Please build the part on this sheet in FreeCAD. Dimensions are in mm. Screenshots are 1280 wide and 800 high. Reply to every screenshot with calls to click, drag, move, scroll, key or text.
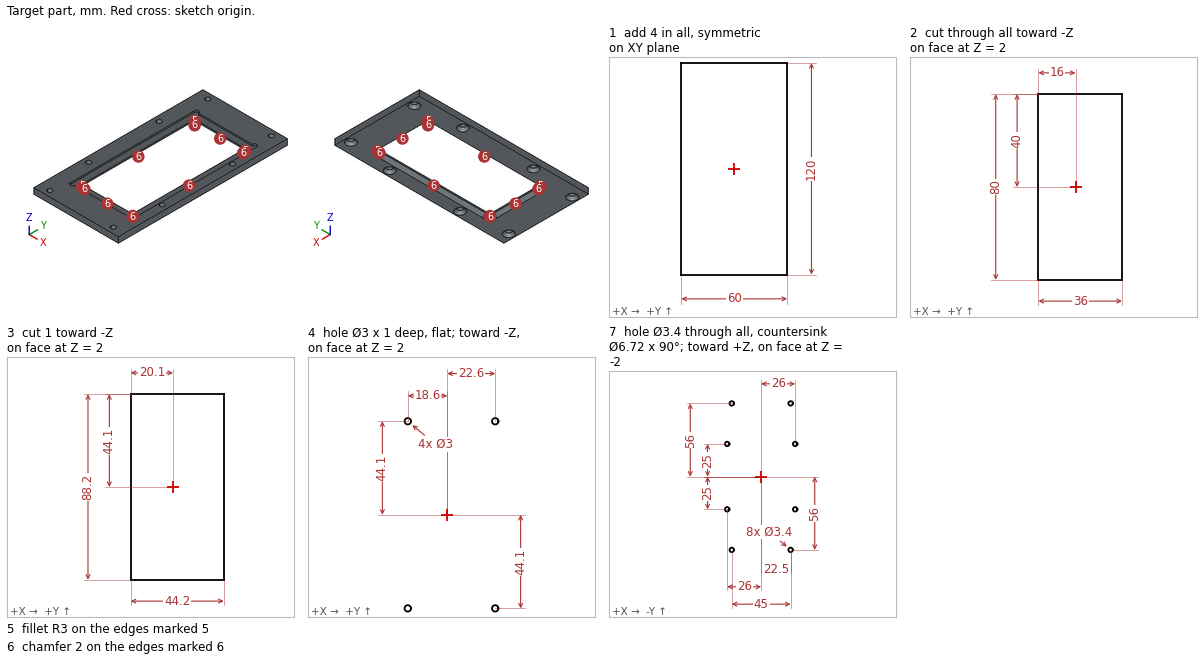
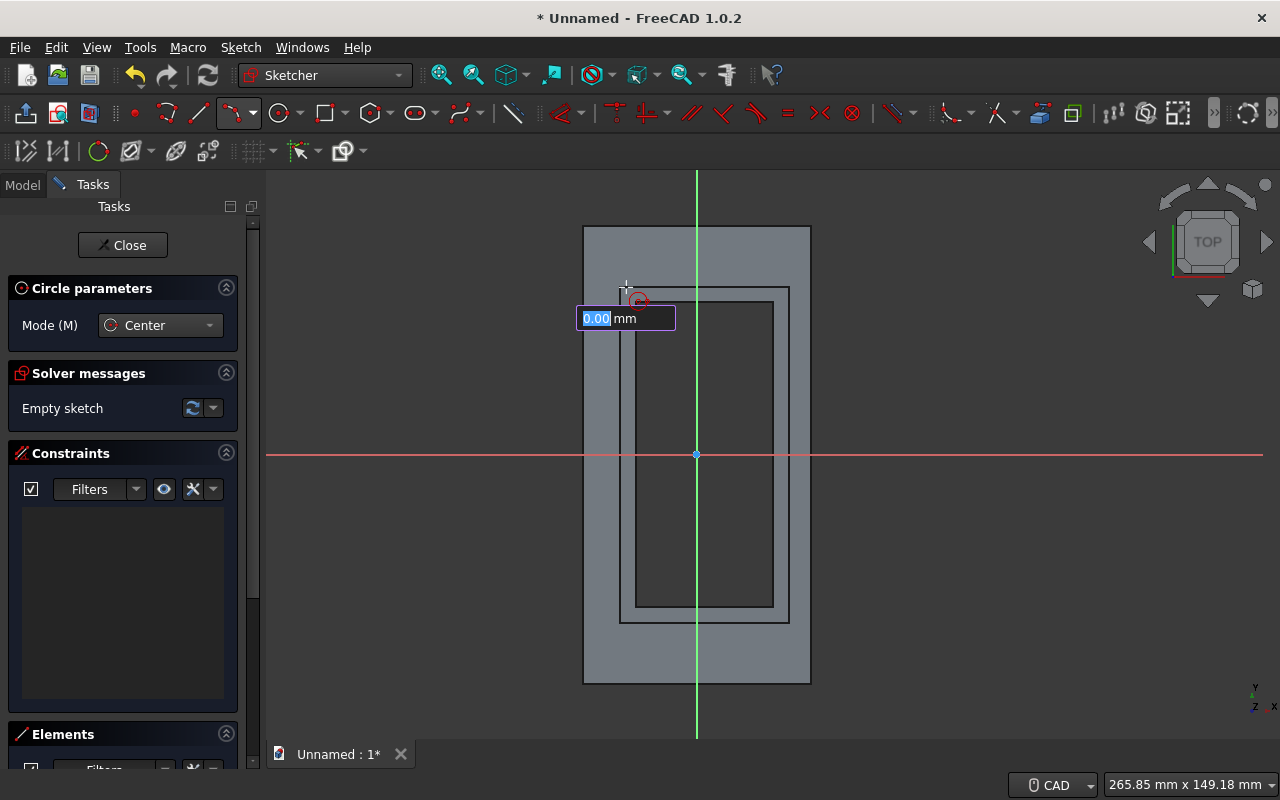
scroll(630, 283, up, 6)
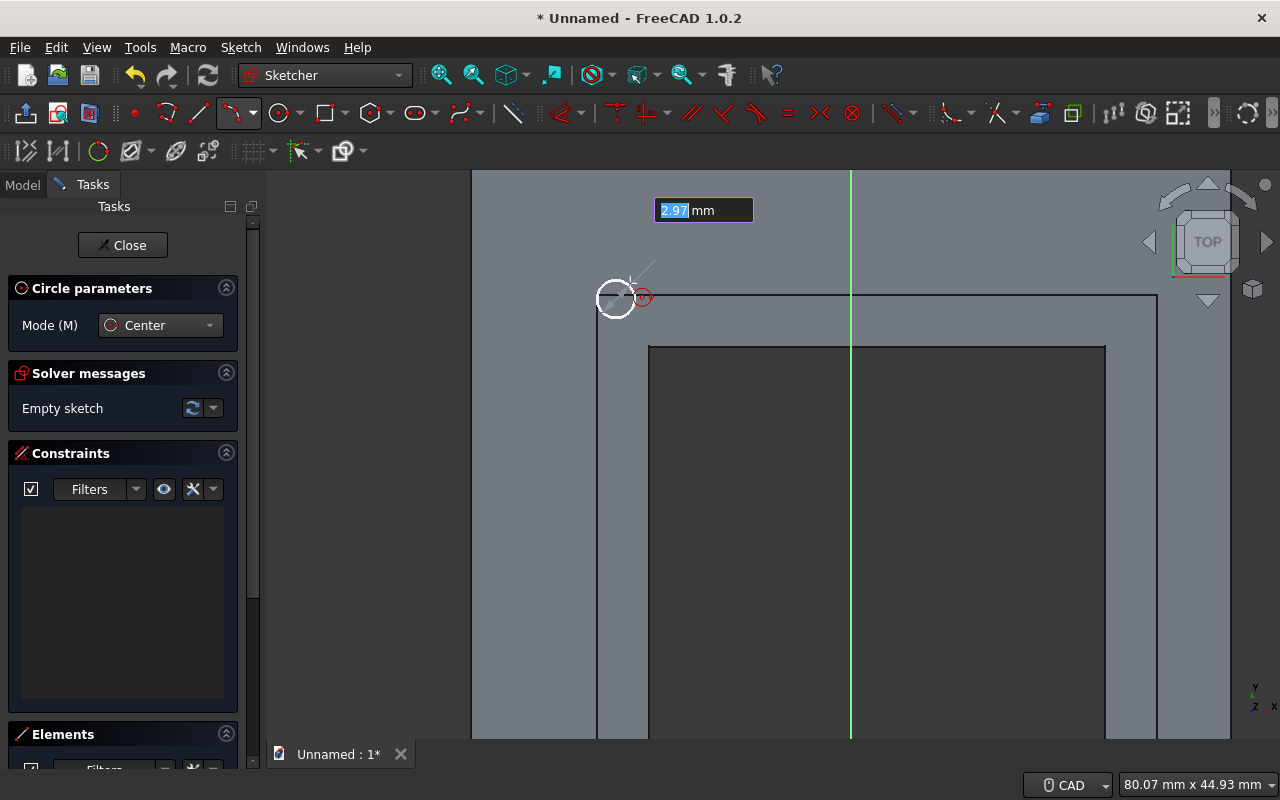
click(629, 281)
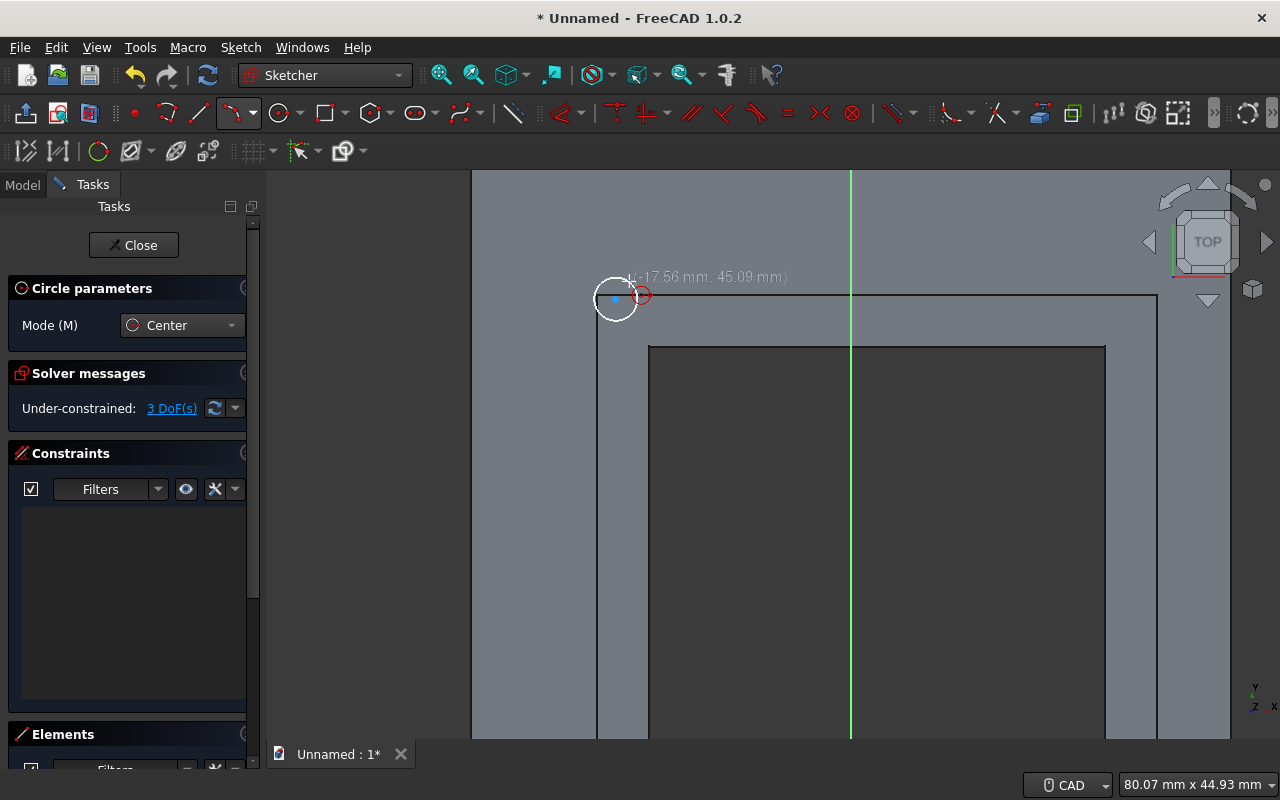
scroll(630, 283, down, 6)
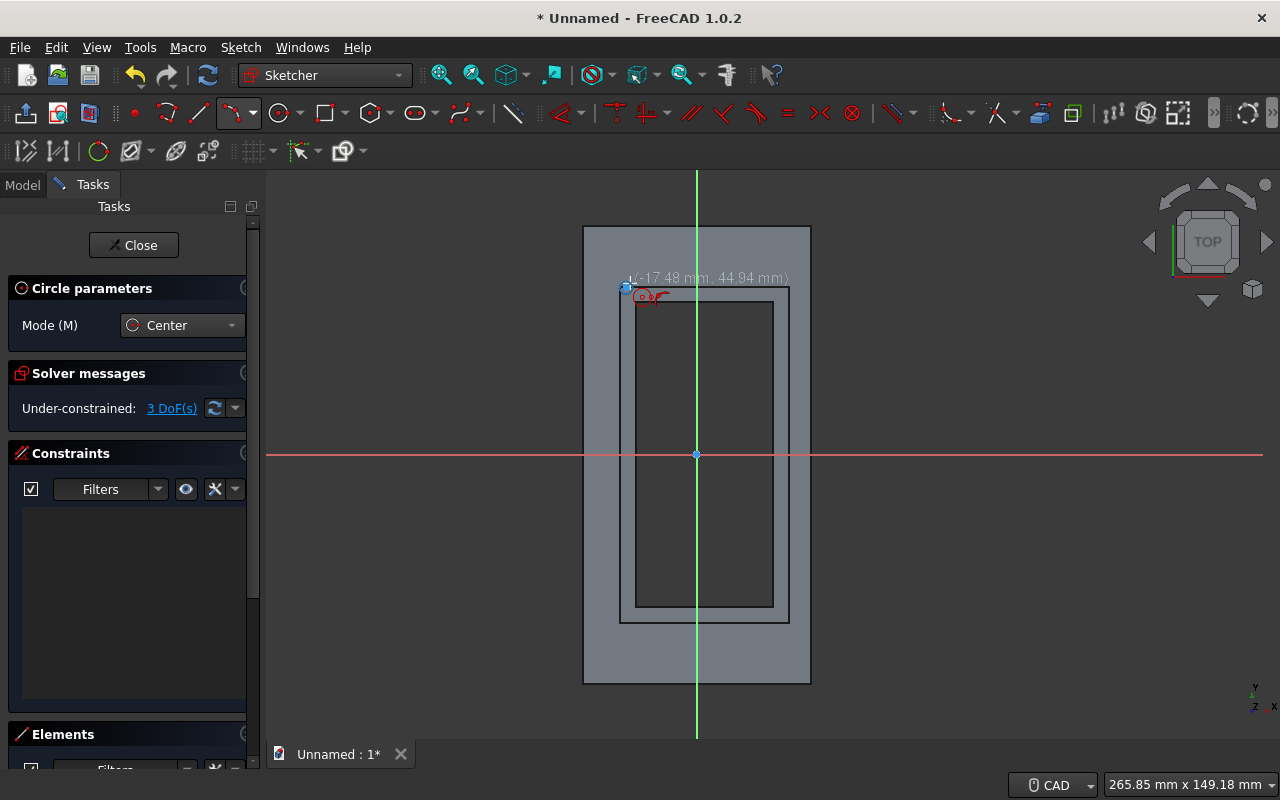
scroll(783, 287, up, 7)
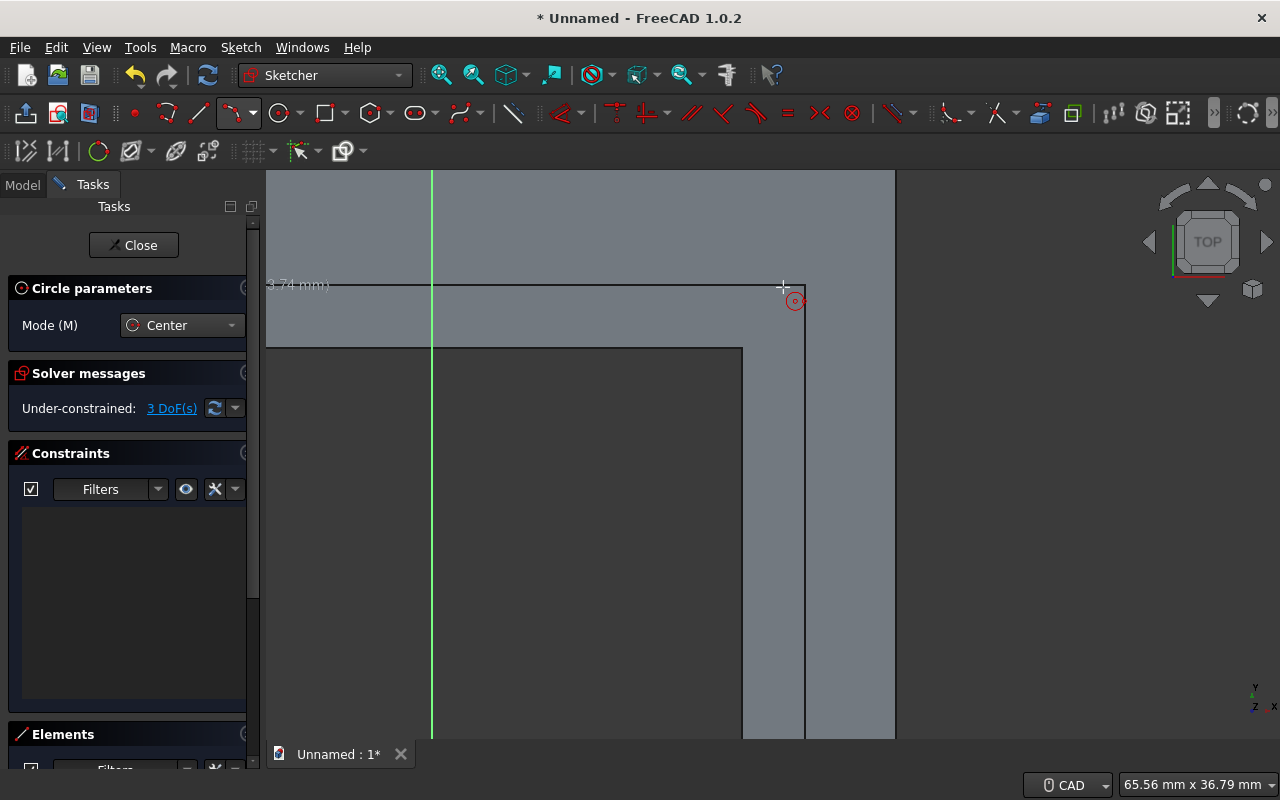
scroll(783, 287, down, 7)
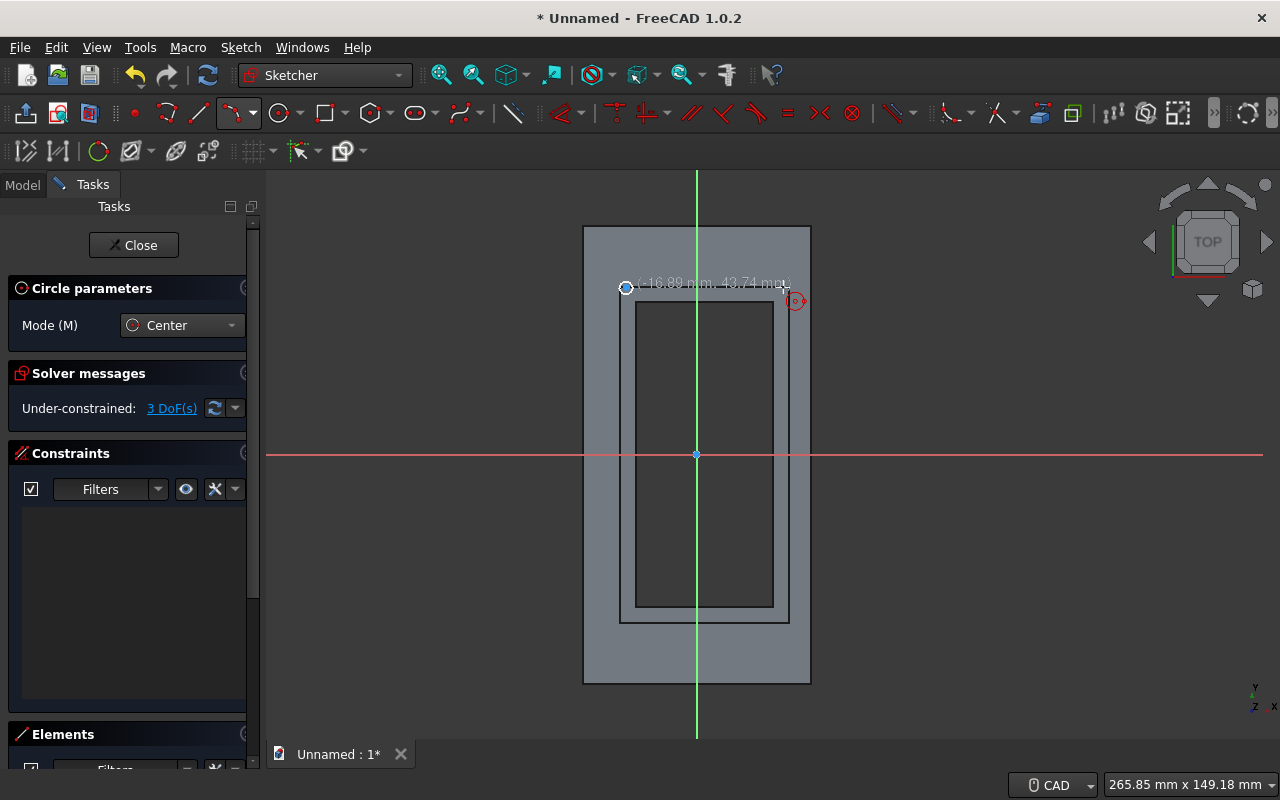
click(783, 287)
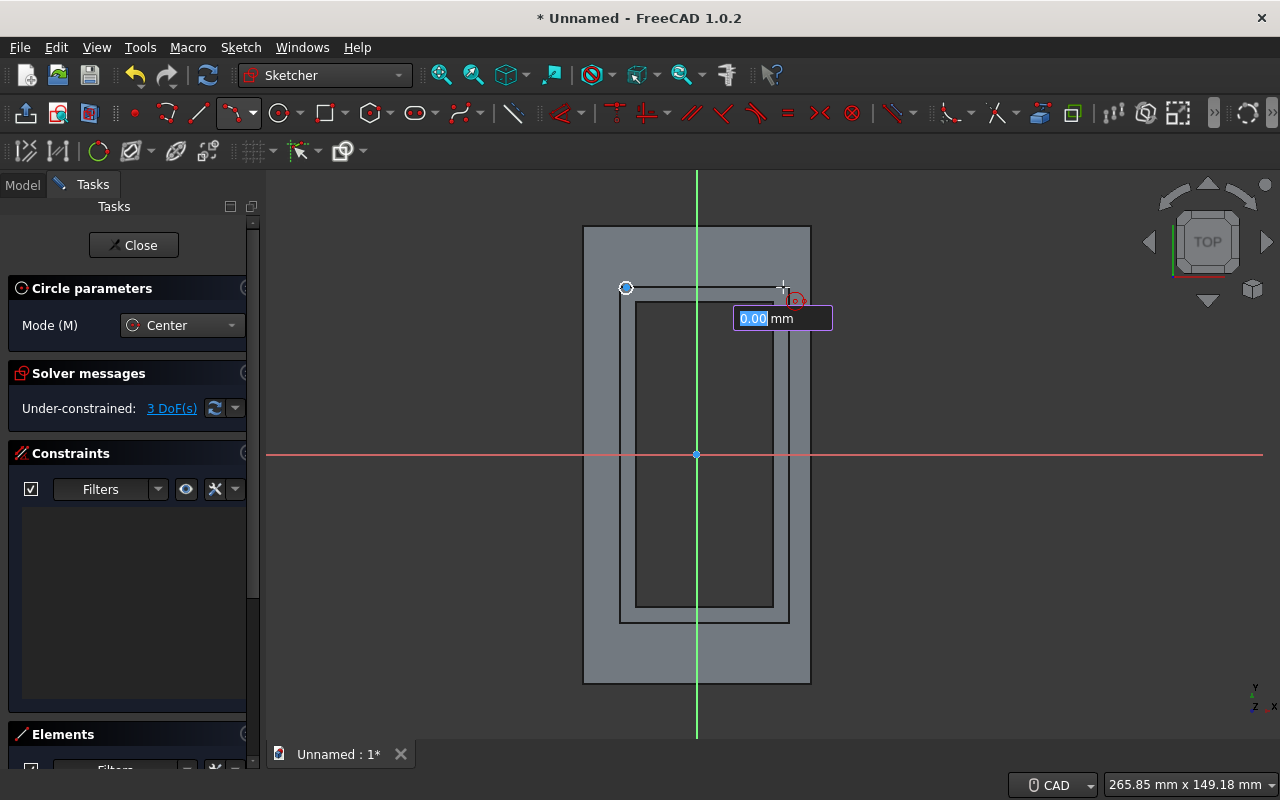
scroll(787, 283, up, 6)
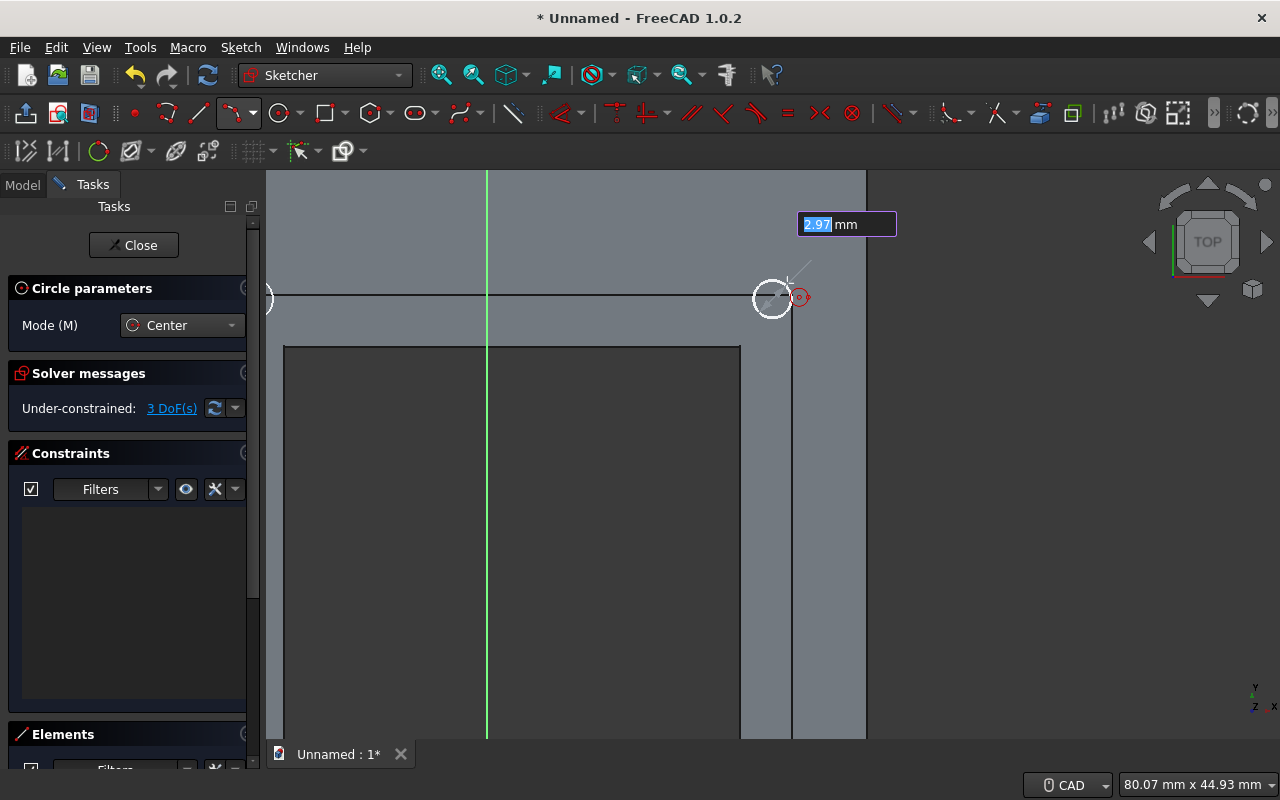
click(786, 281)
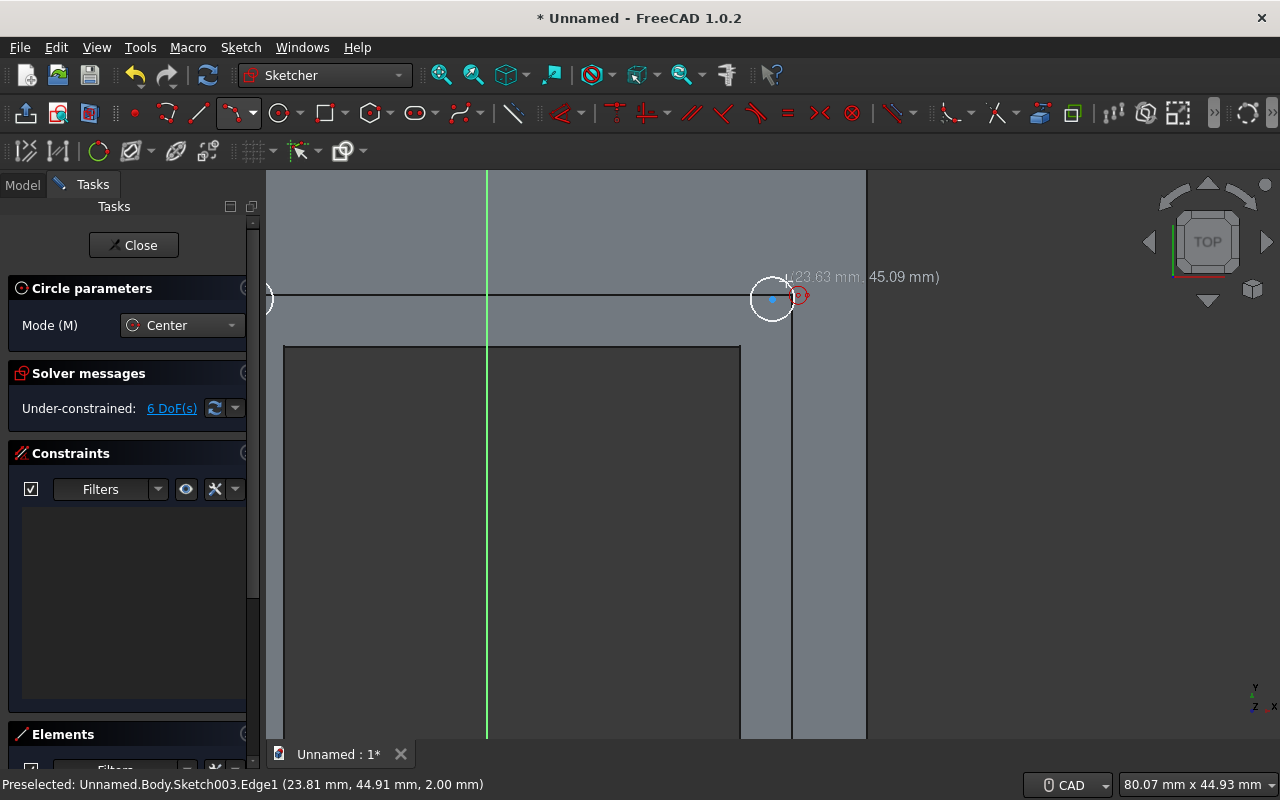
scroll(787, 283, down, 6)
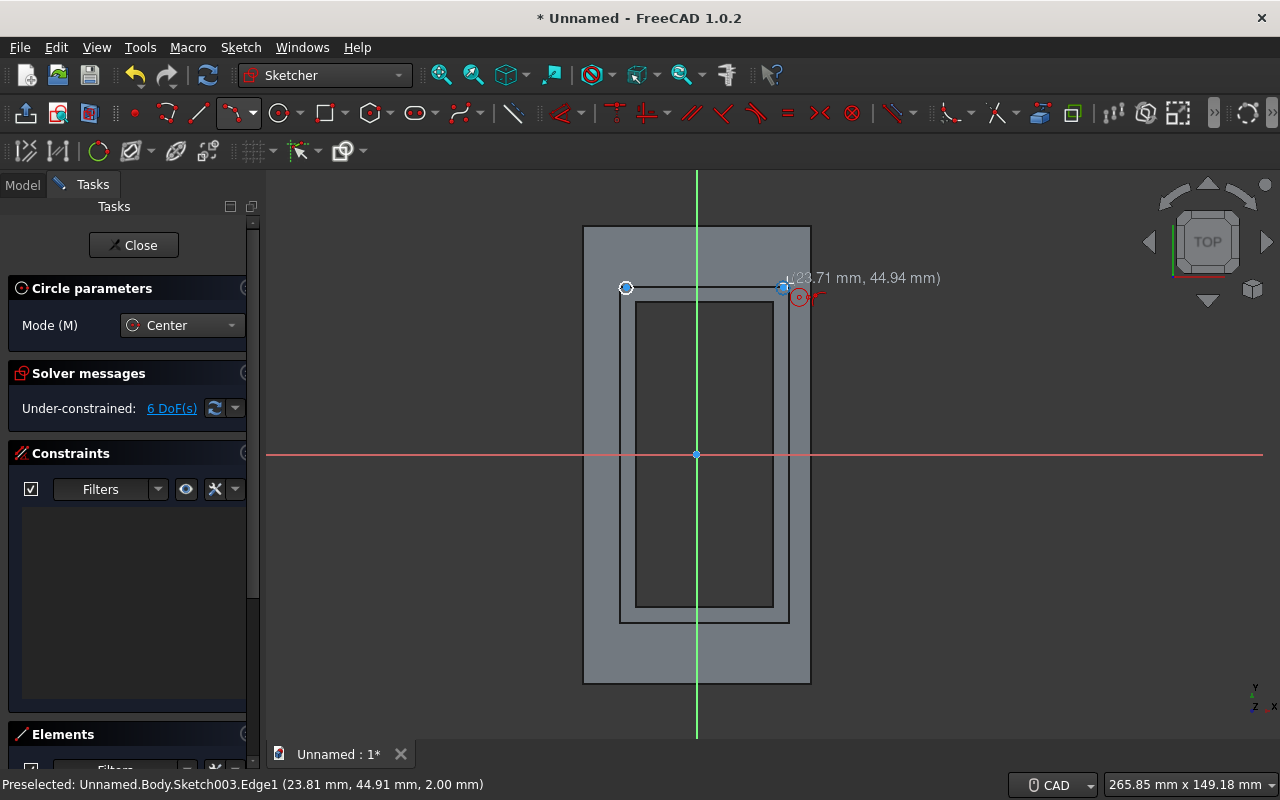
scroll(783, 623, up, 7)